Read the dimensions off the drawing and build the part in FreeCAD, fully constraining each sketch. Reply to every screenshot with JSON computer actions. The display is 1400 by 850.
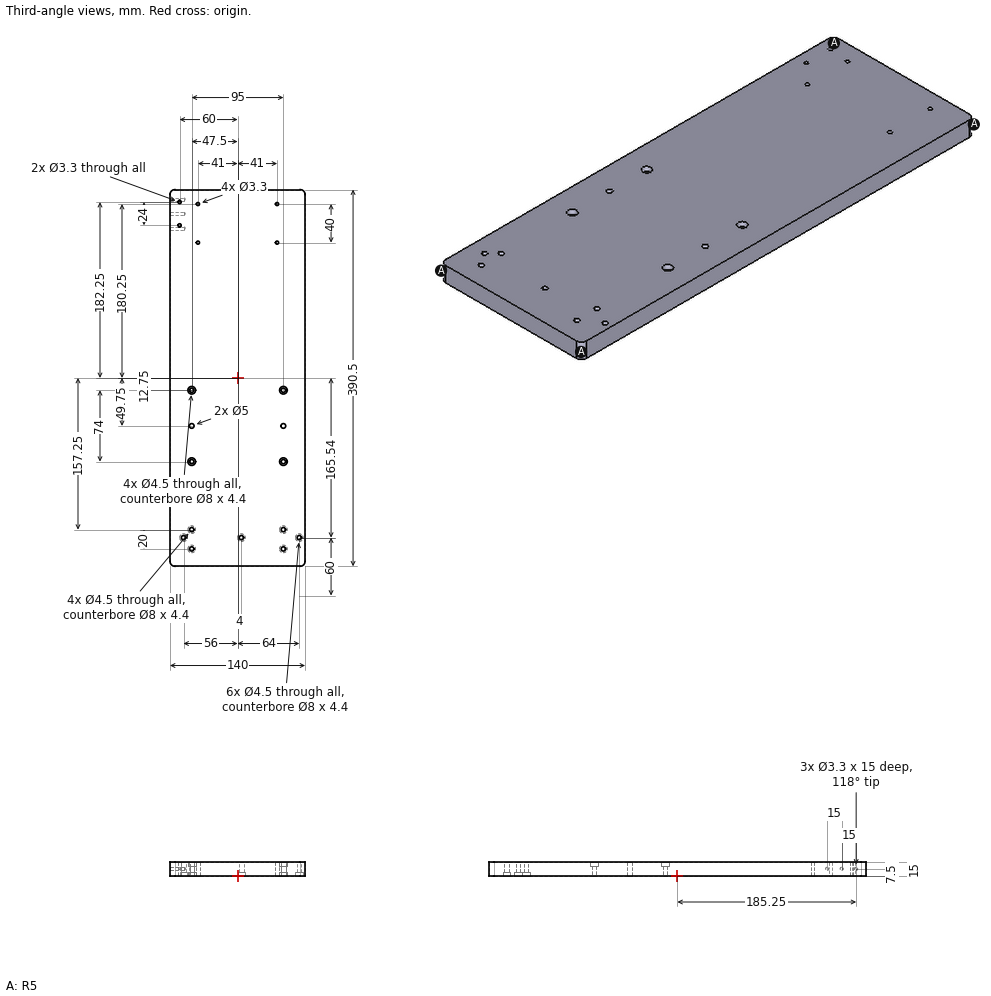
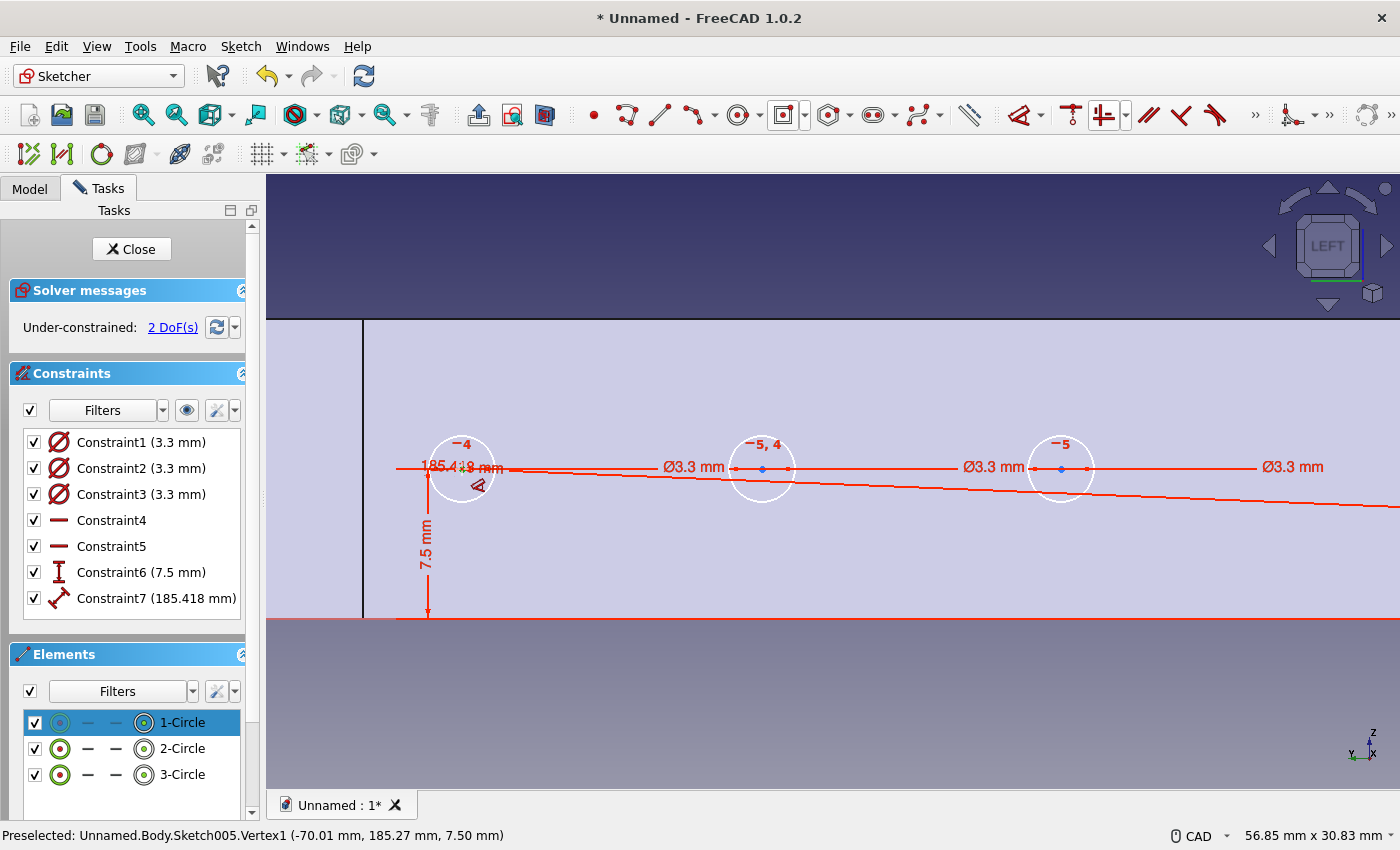
{"action": "left_click", "coordinate": [762, 469]}
{"action": "left_click", "coordinate": [612, 503]}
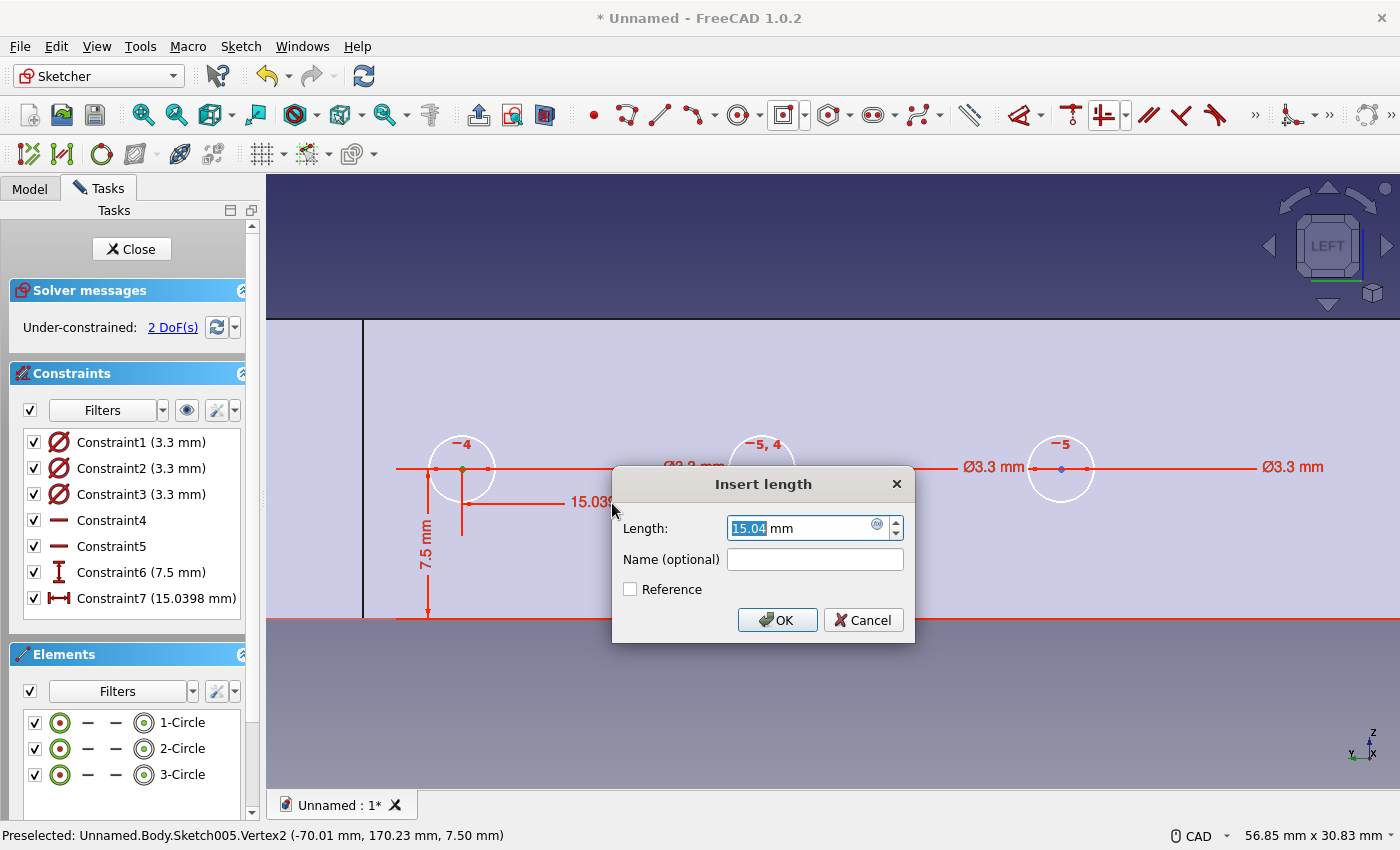
{"action": "type", "text": "15"}
{"action": "key", "text": "Return"}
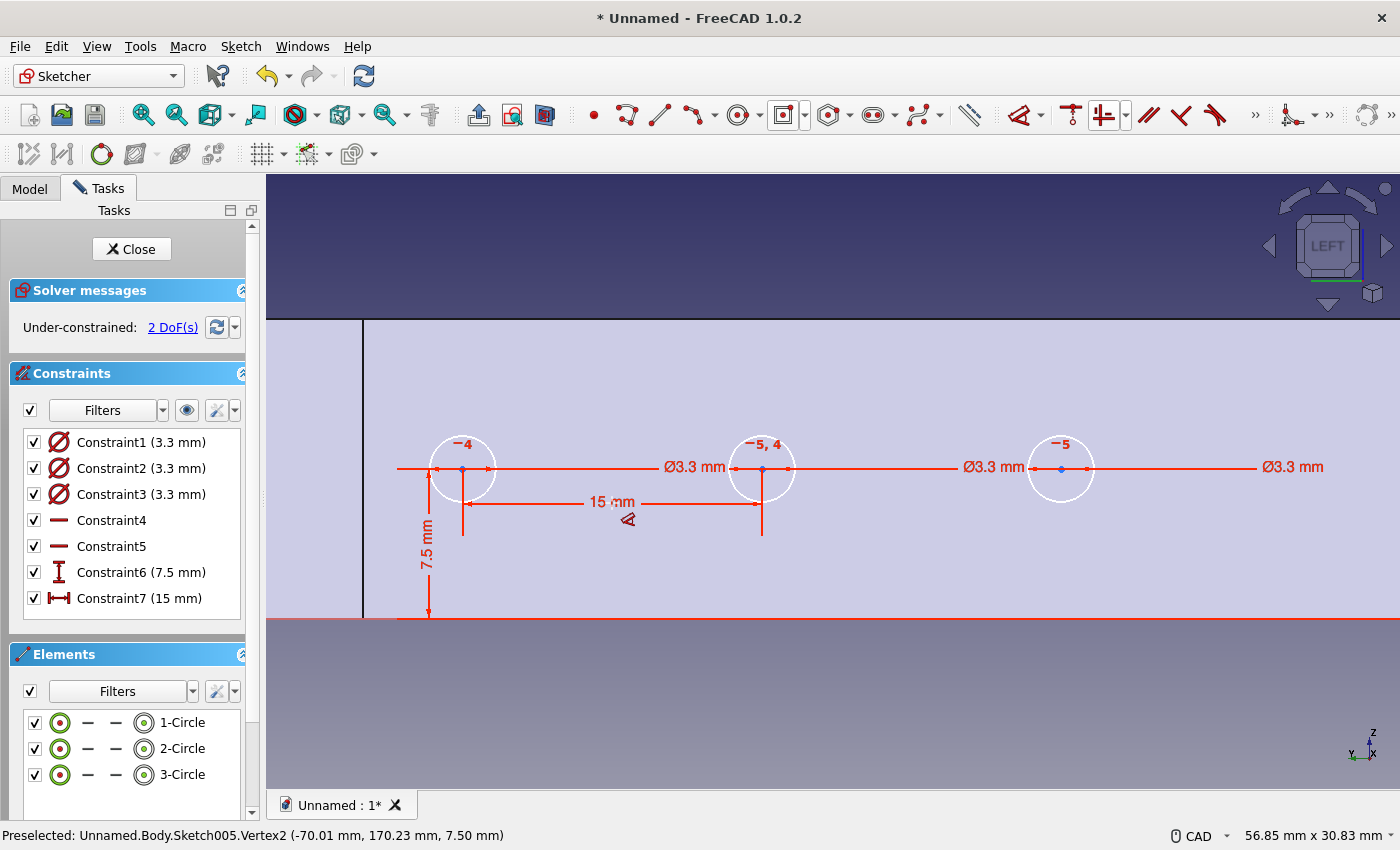
{"action": "left_click", "coordinate": [762, 469]}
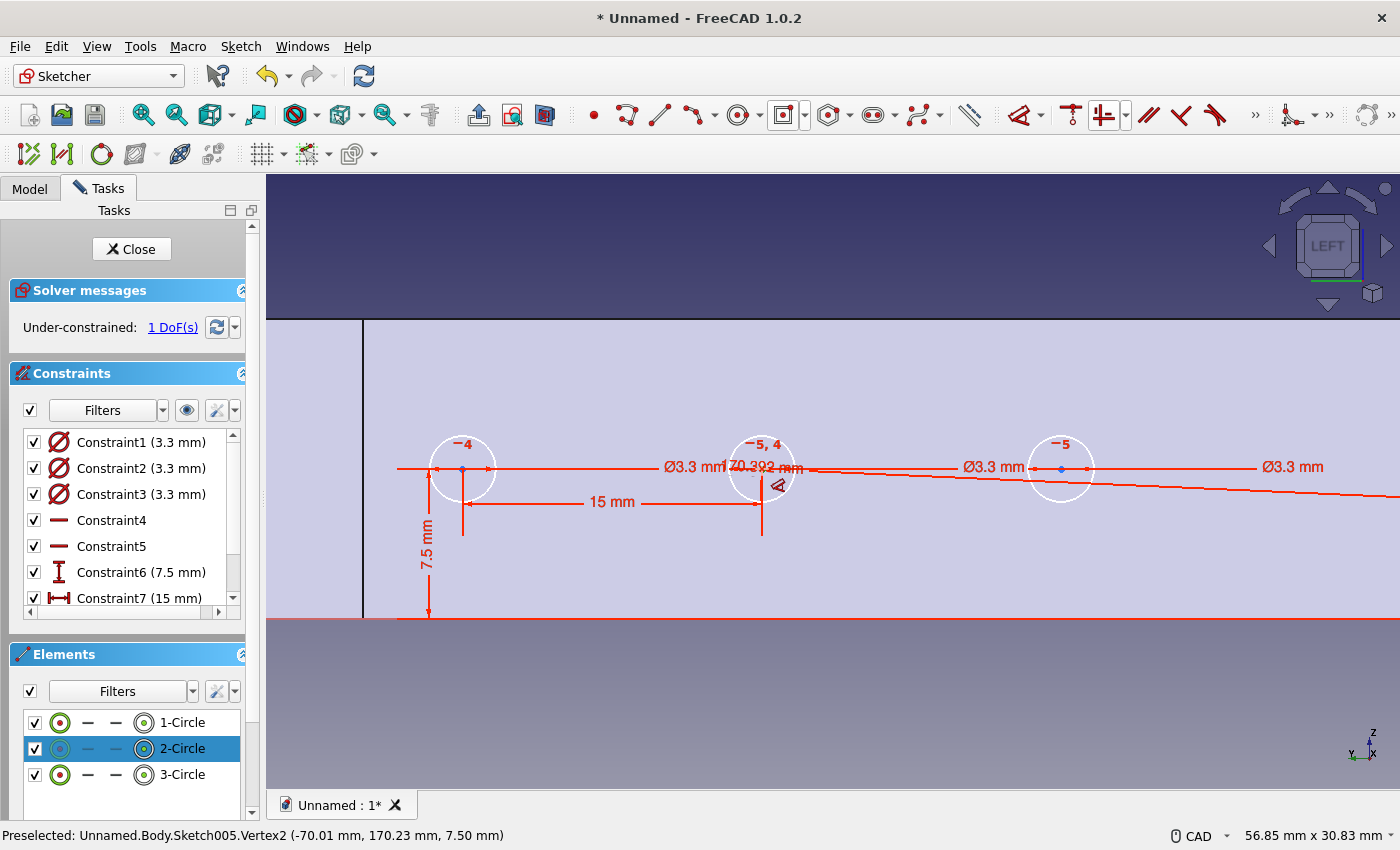
{"action": "left_click", "coordinate": [1061, 469]}
{"action": "left_click", "coordinate": [911, 503]}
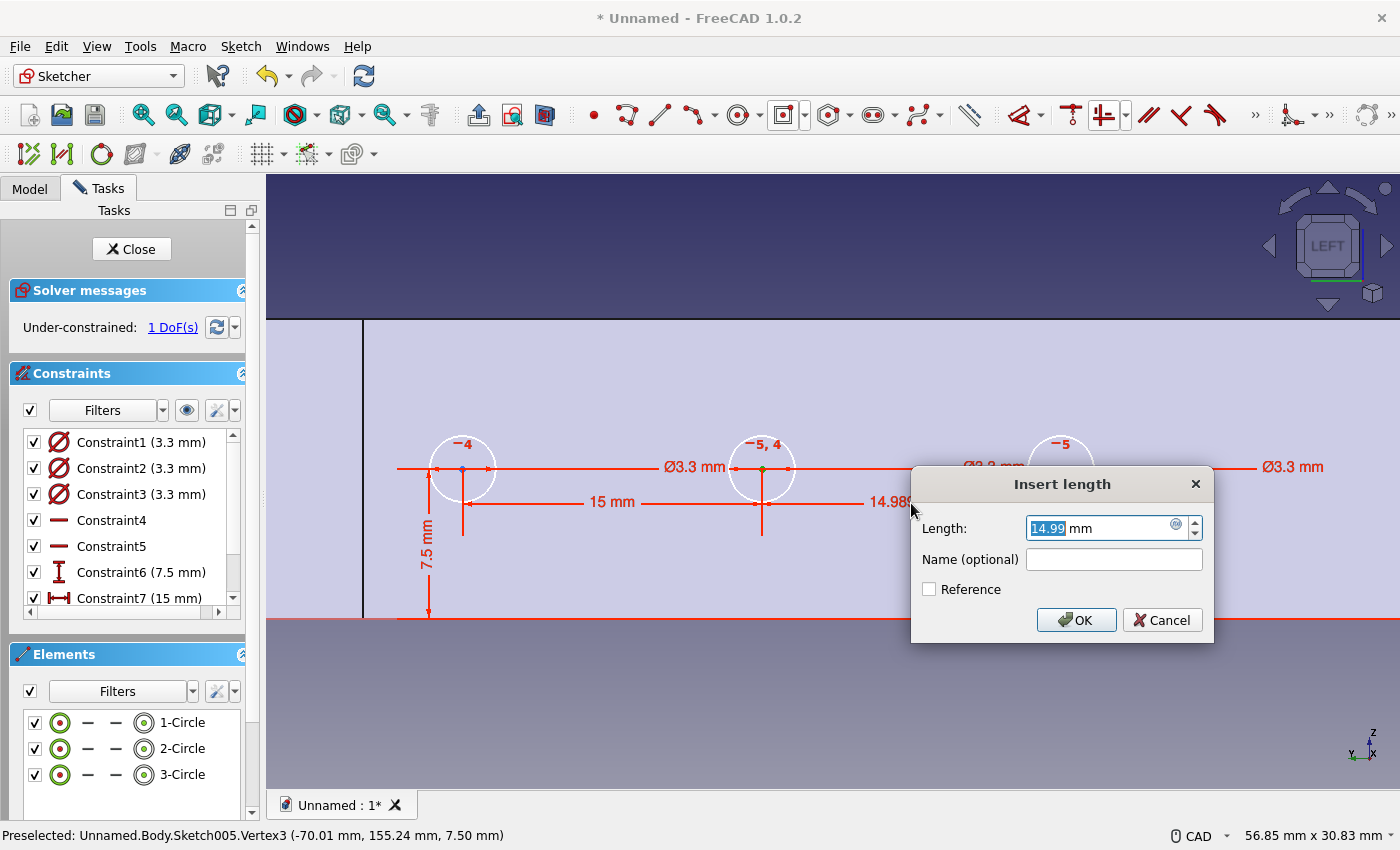
{"action": "type", "text": "15"}
{"action": "key", "text": "Return"}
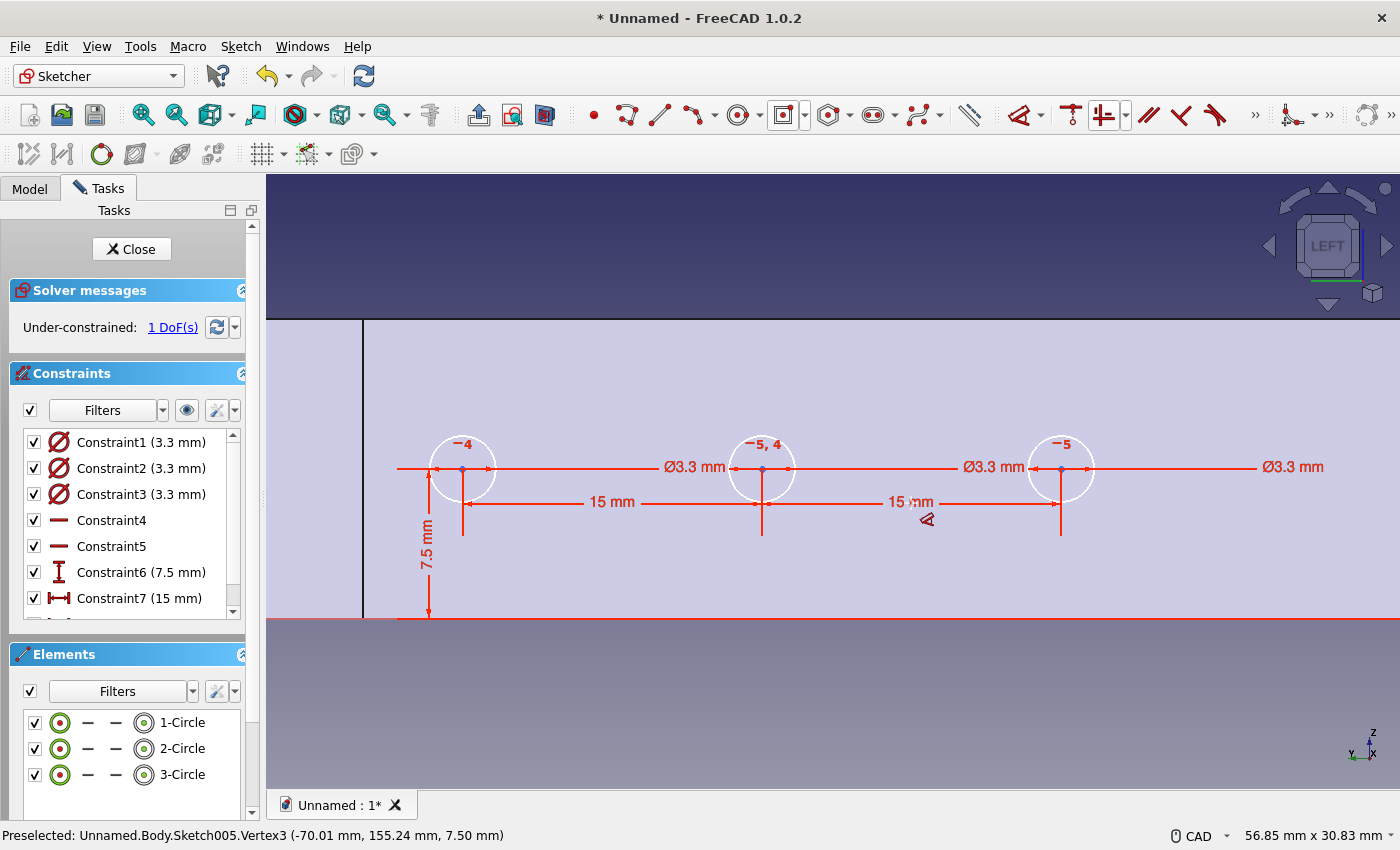
{"action": "left_click", "coordinate": [463, 469]}
{"action": "left_click", "coordinate": [849, 653]}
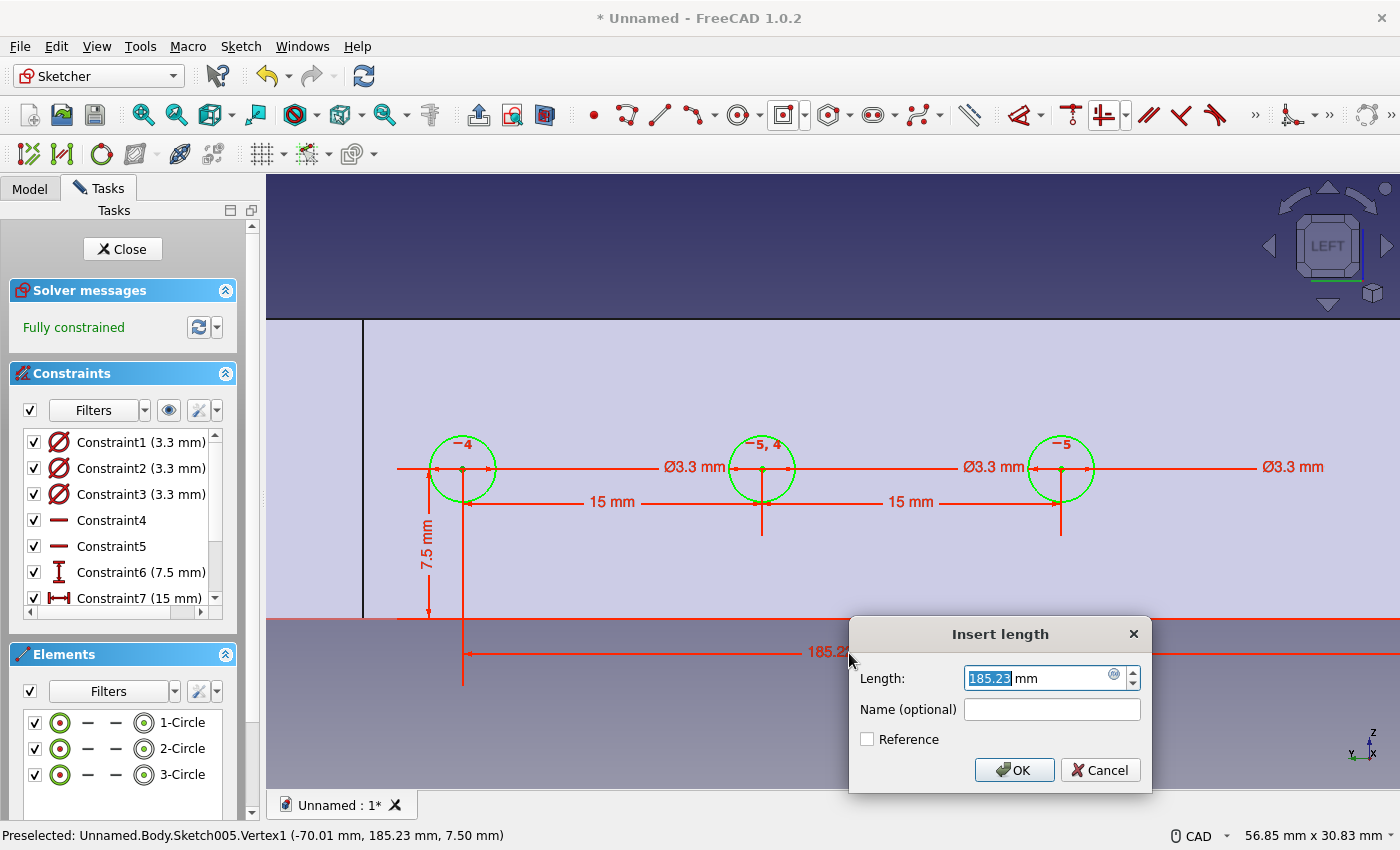
{"action": "type", "text": "185.25"}
{"action": "key", "text": "Return"}
{"action": "key", "text": "Escape"}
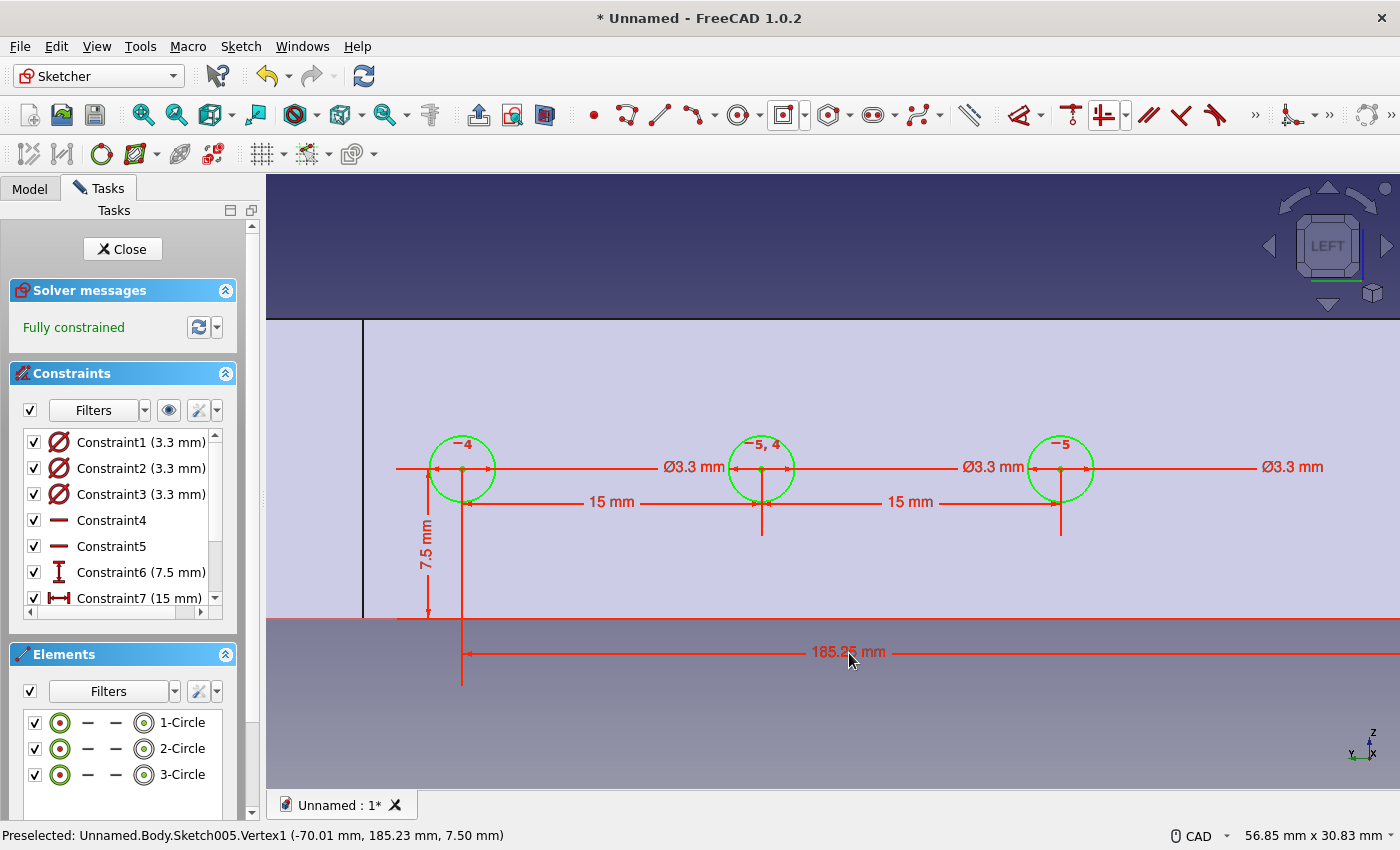
{"action": "left_click", "coordinate": [123, 249]}